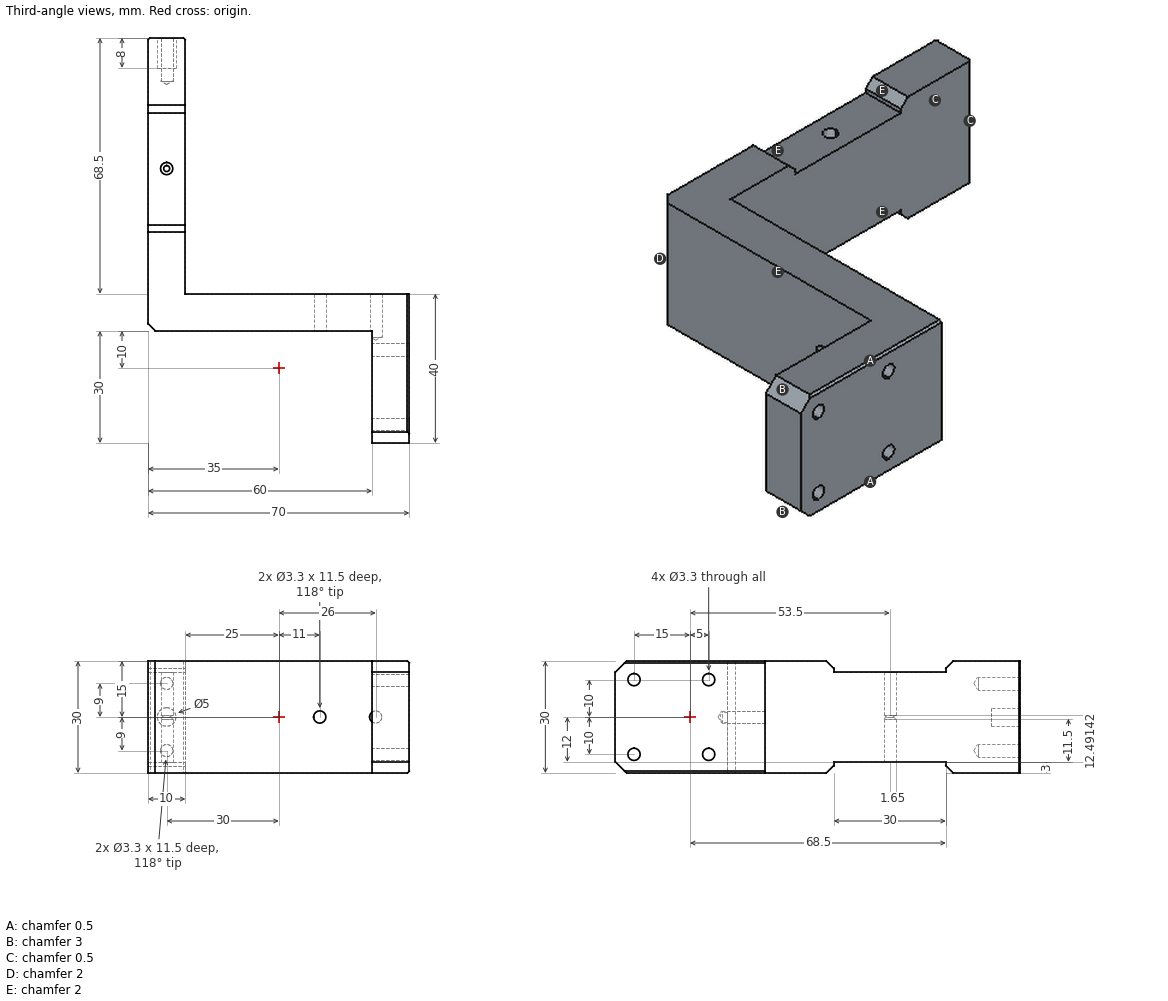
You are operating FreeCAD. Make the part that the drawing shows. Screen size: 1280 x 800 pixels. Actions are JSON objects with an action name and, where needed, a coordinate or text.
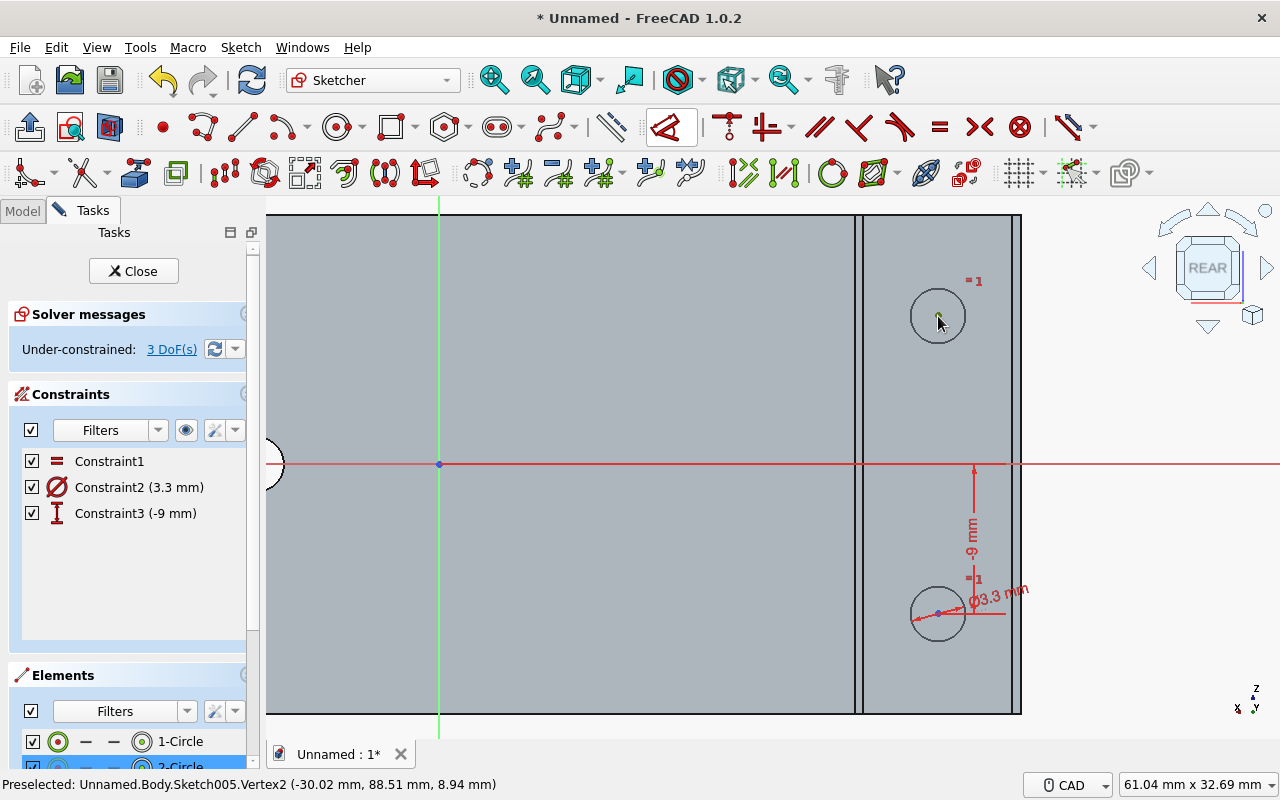
{"action": "left_click", "coordinate": [692, 128]}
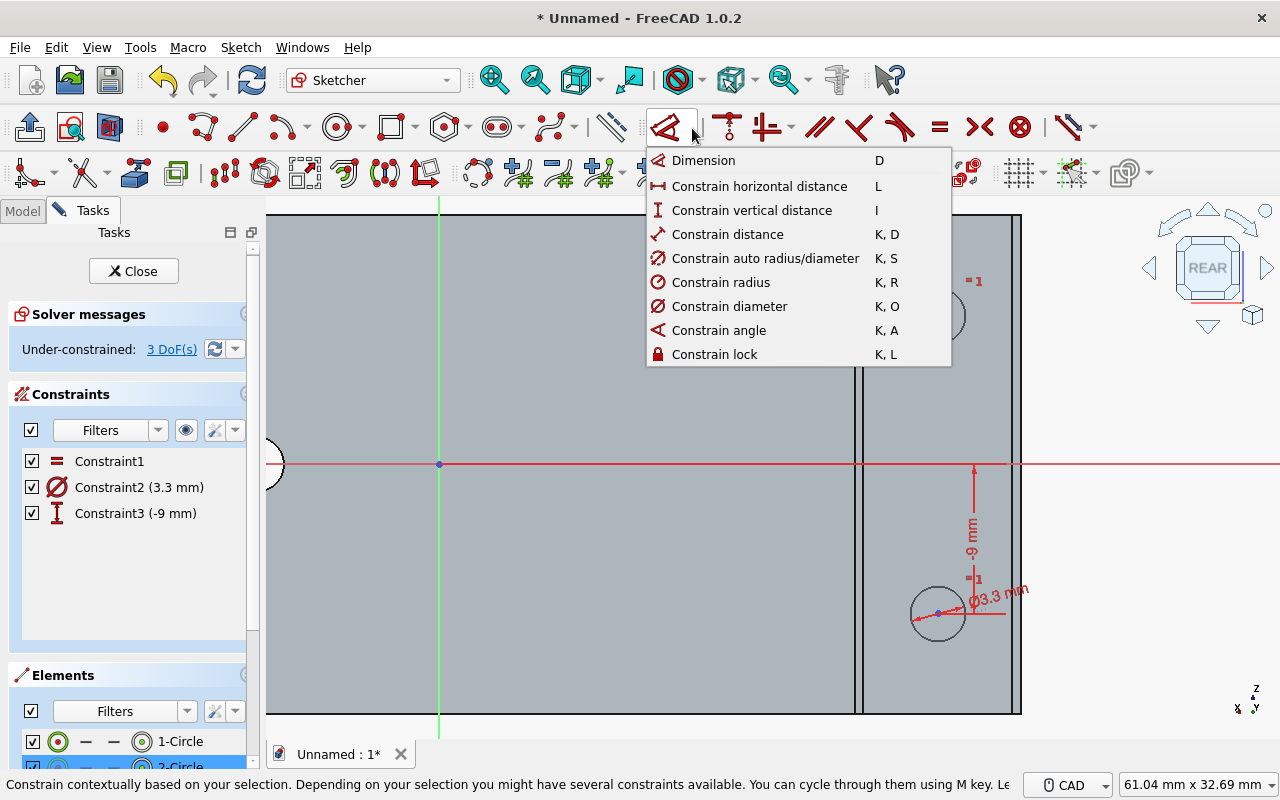
{"action": "left_click", "coordinate": [799, 210]}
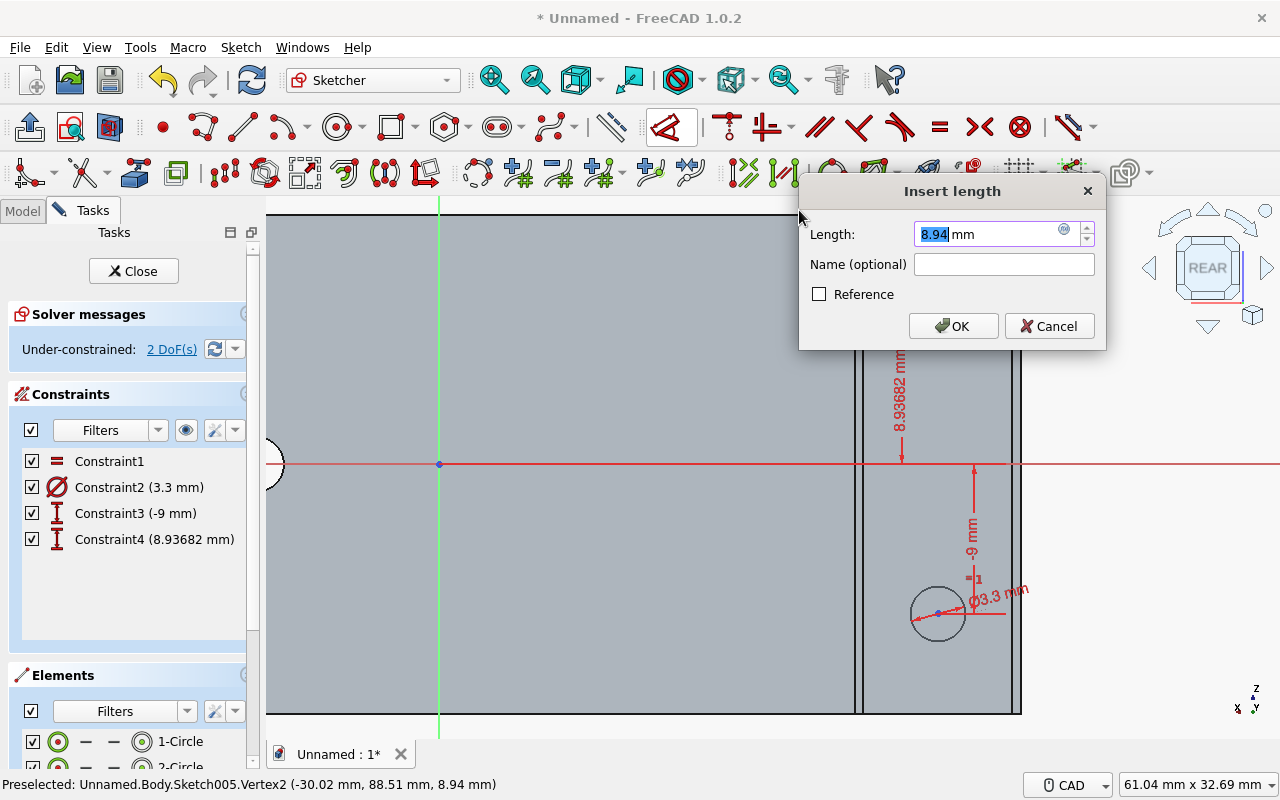
{"action": "type", "text": "9"}
{"action": "key", "text": "Return"}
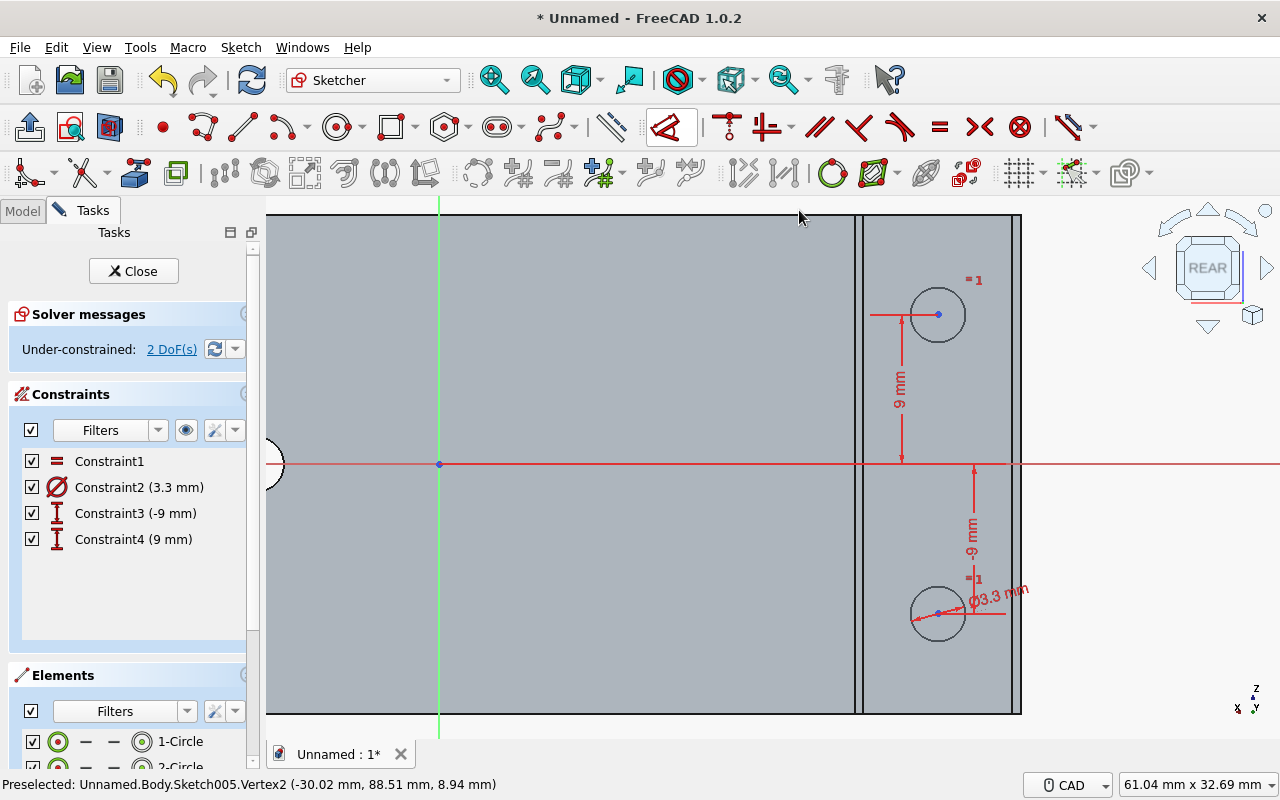
{"action": "left_click", "coordinate": [938, 614]}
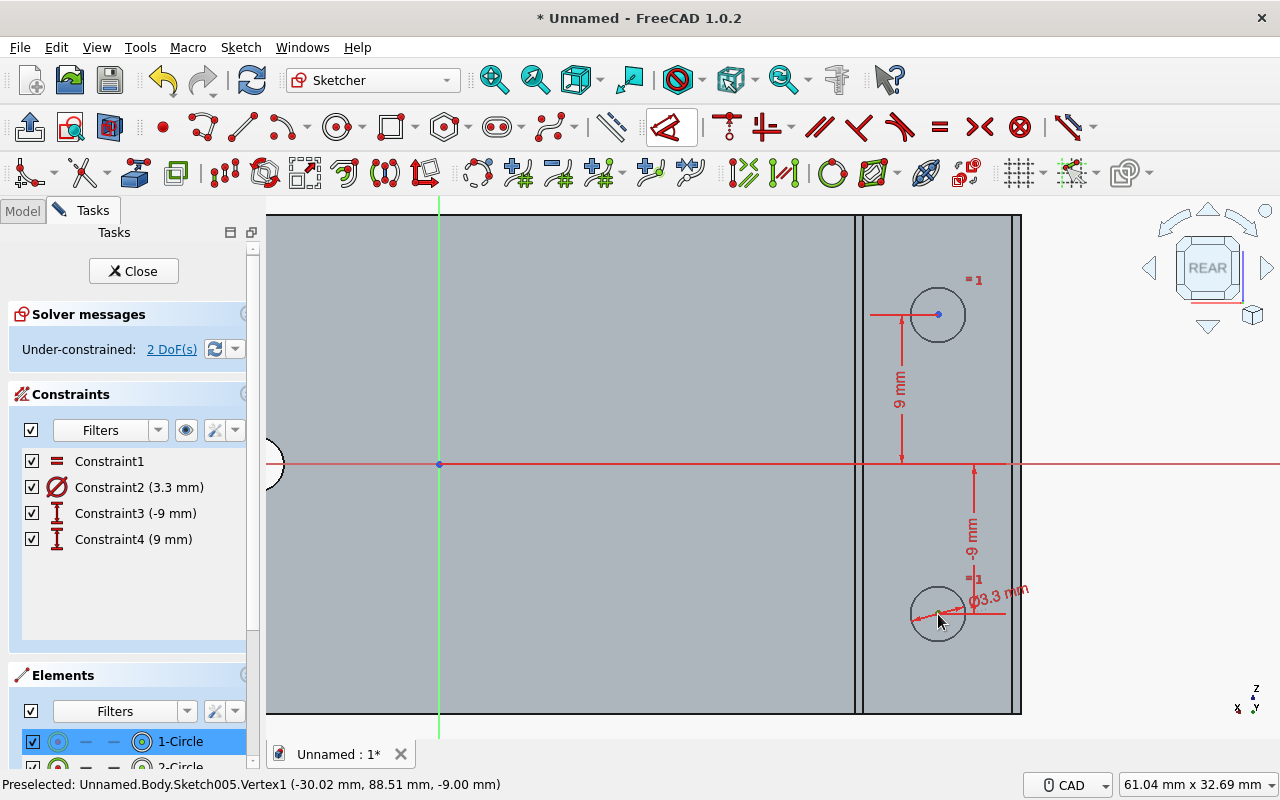
{"action": "key", "text": "l"}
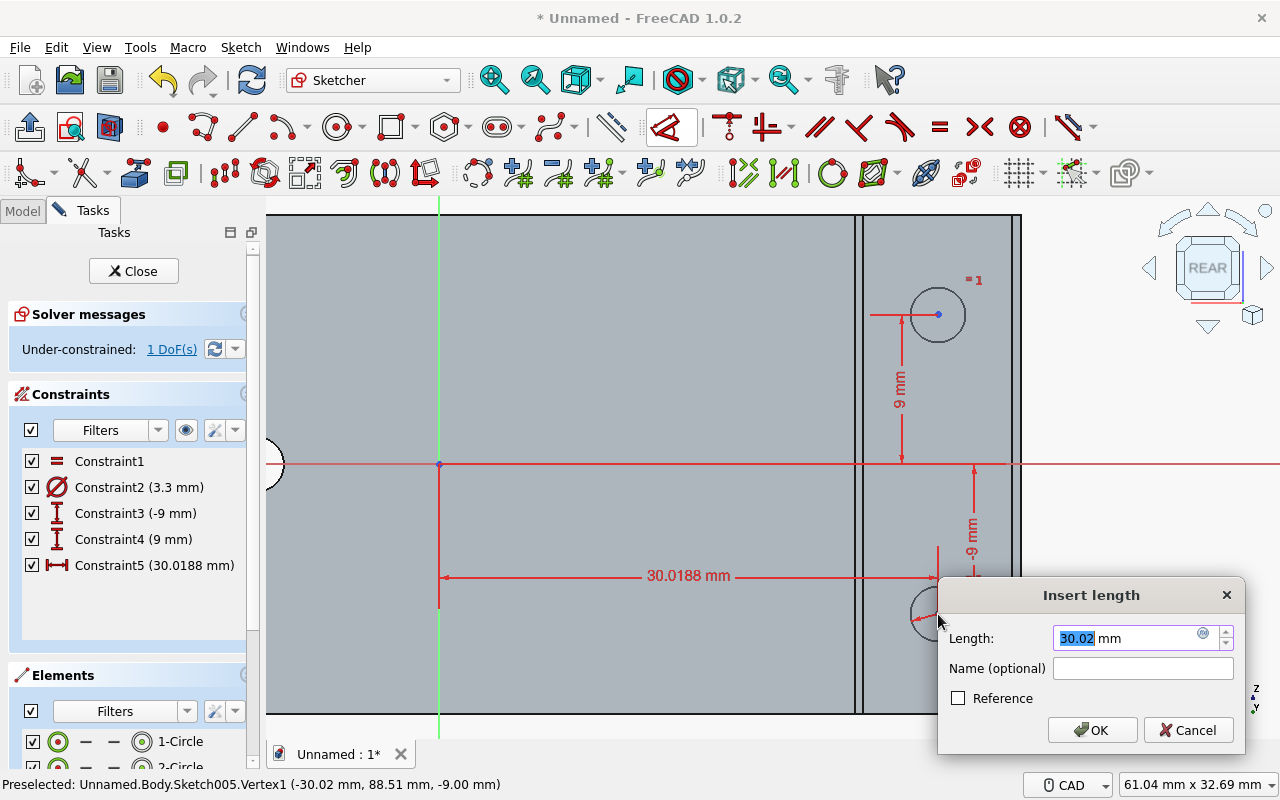
{"action": "type", "text": "30"}
{"action": "key", "text": "Return"}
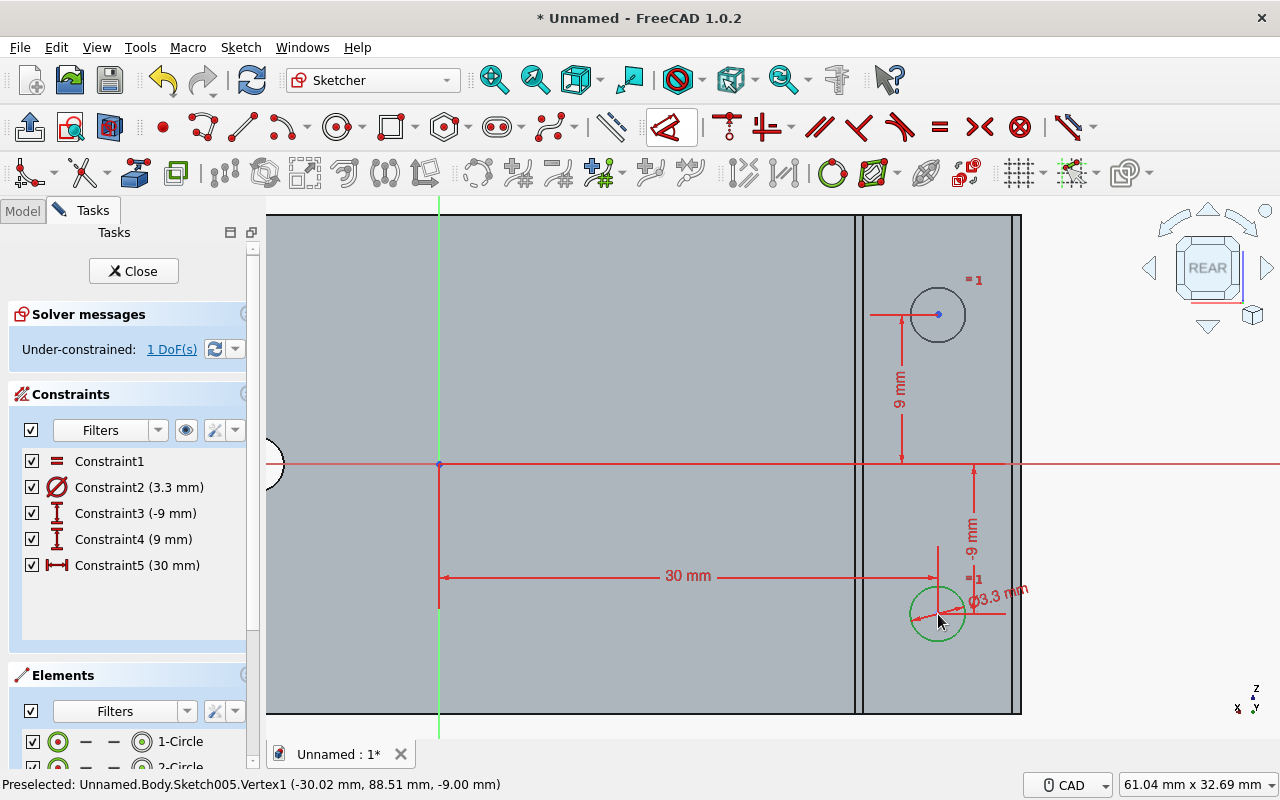
{"action": "left_click", "coordinate": [938, 315]}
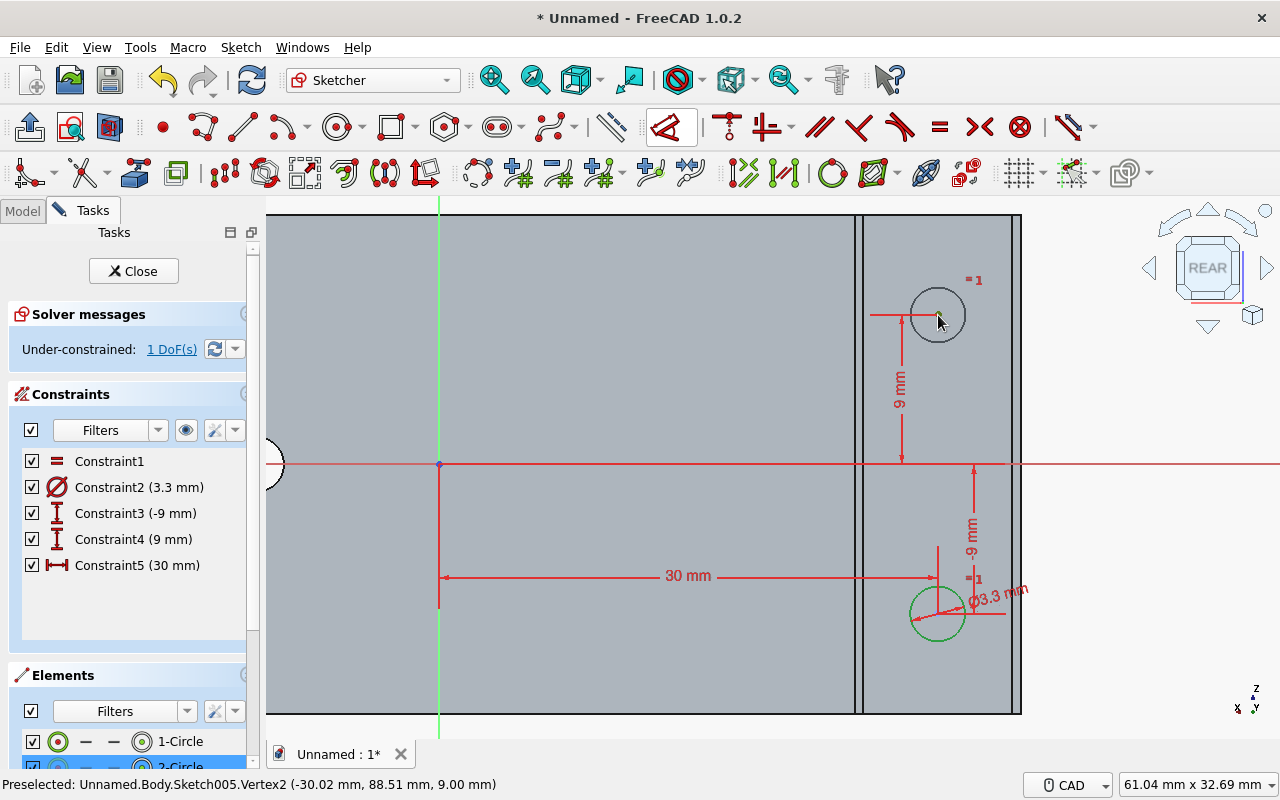
{"action": "left_click", "coordinate": [692, 128]}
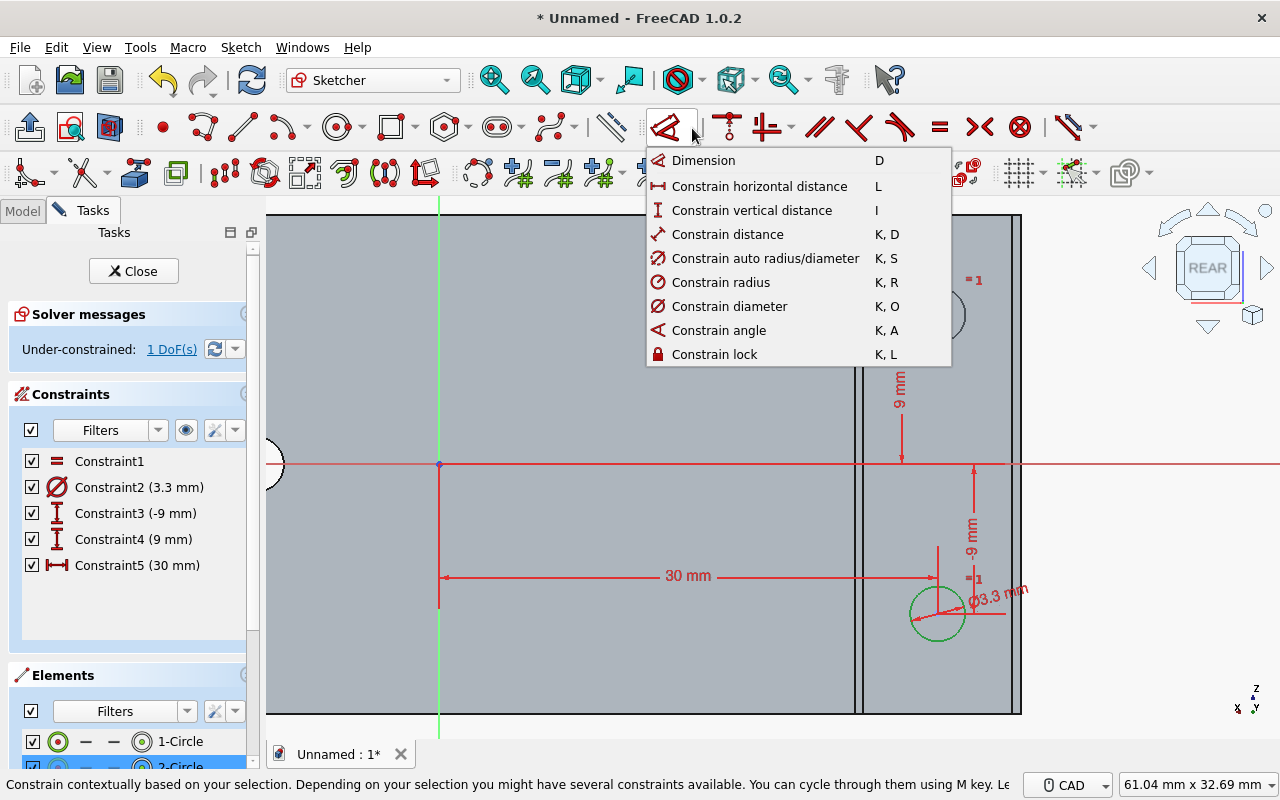
{"action": "left_click", "coordinate": [799, 186]}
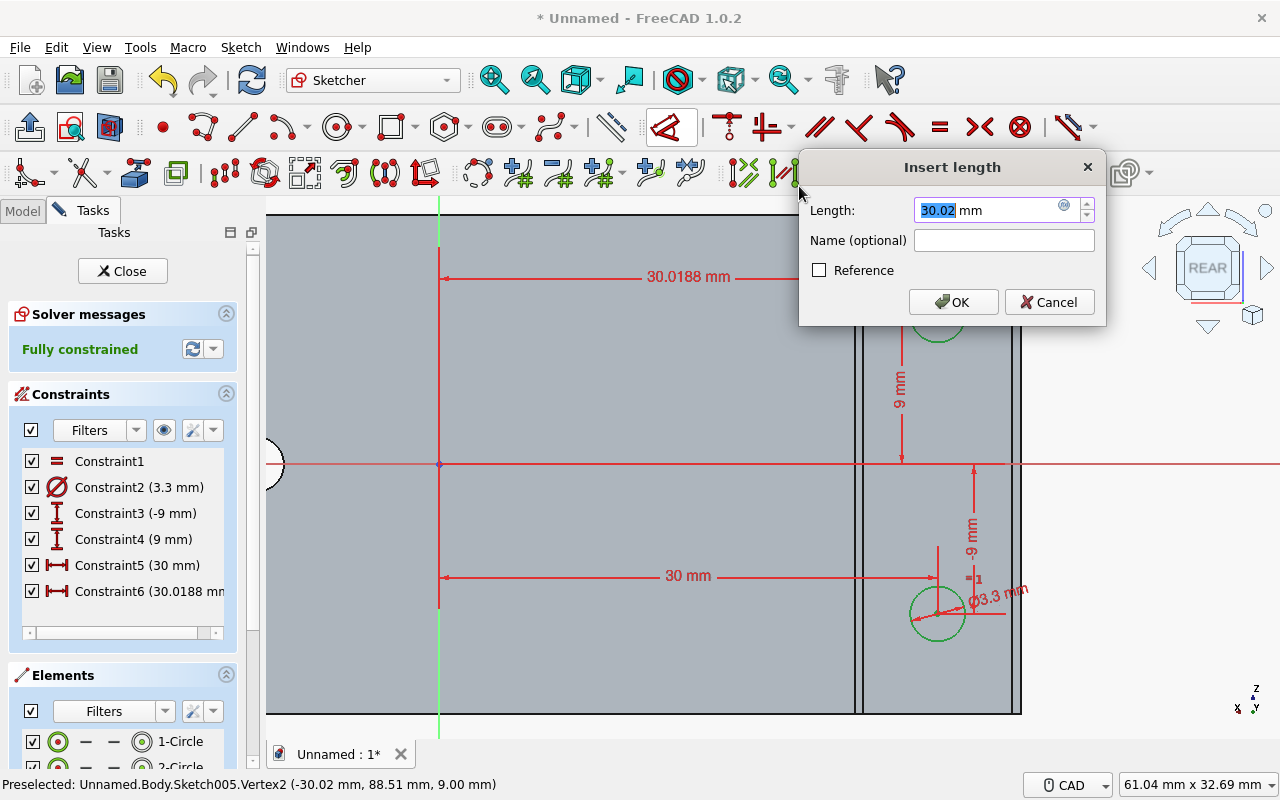
{"action": "type", "text": "30"}
{"action": "key", "text": "Return"}